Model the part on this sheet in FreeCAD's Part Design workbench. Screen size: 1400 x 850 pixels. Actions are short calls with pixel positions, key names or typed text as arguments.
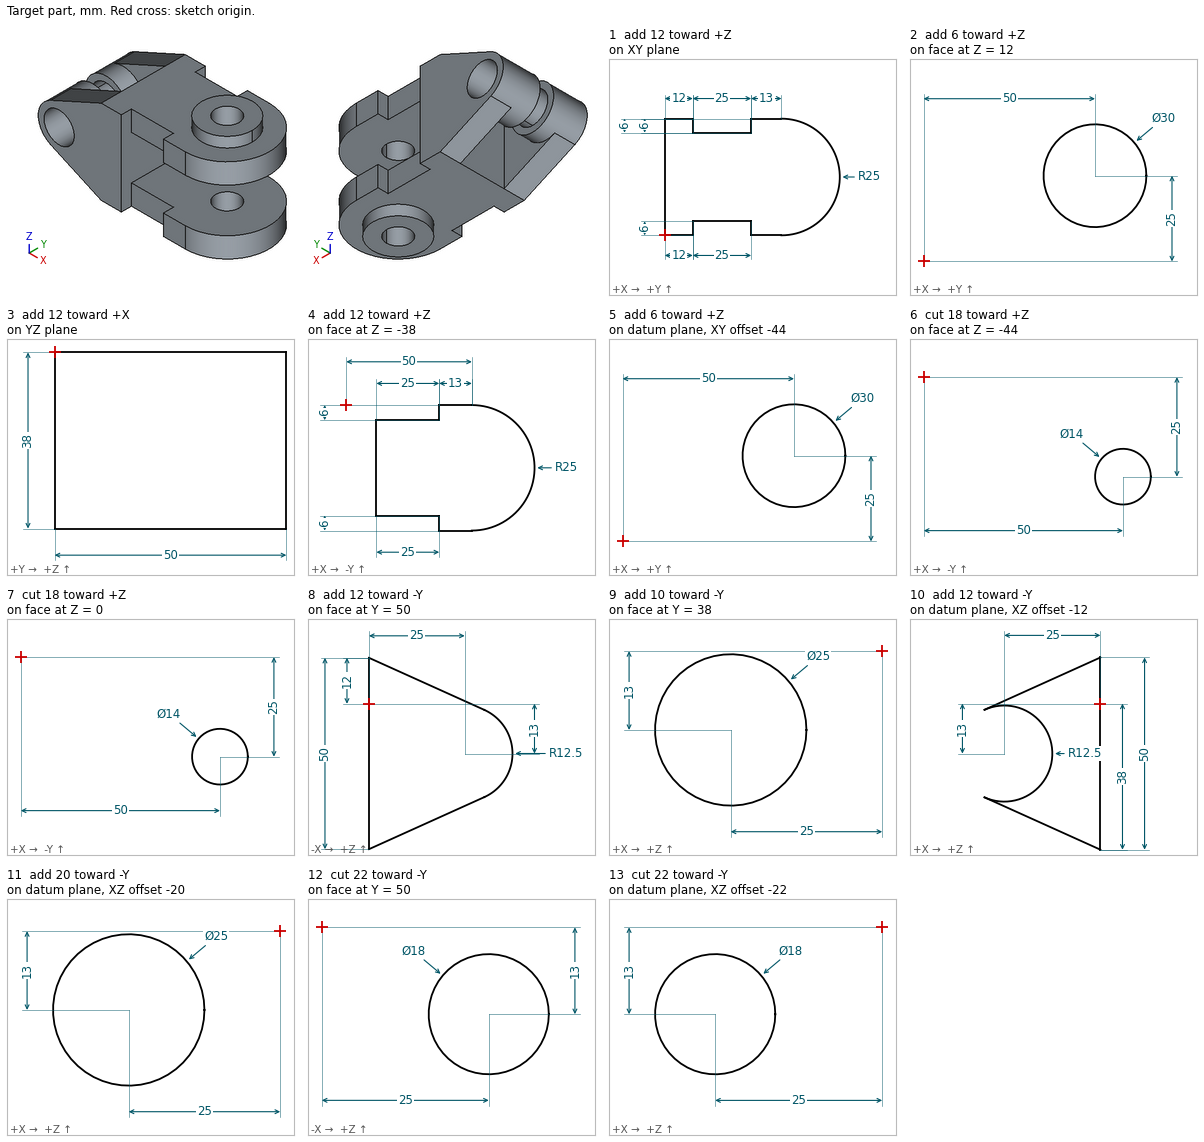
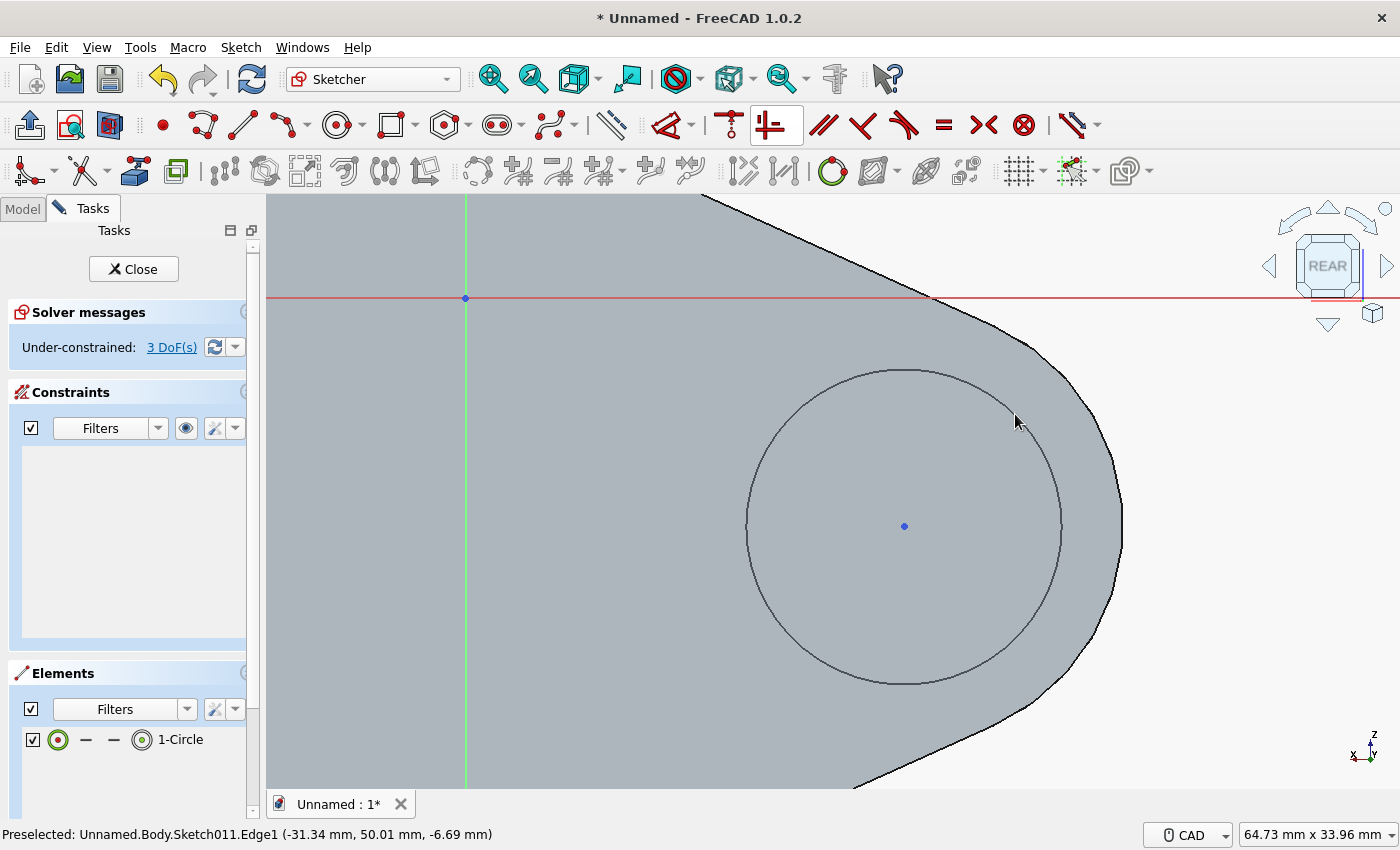
key(d)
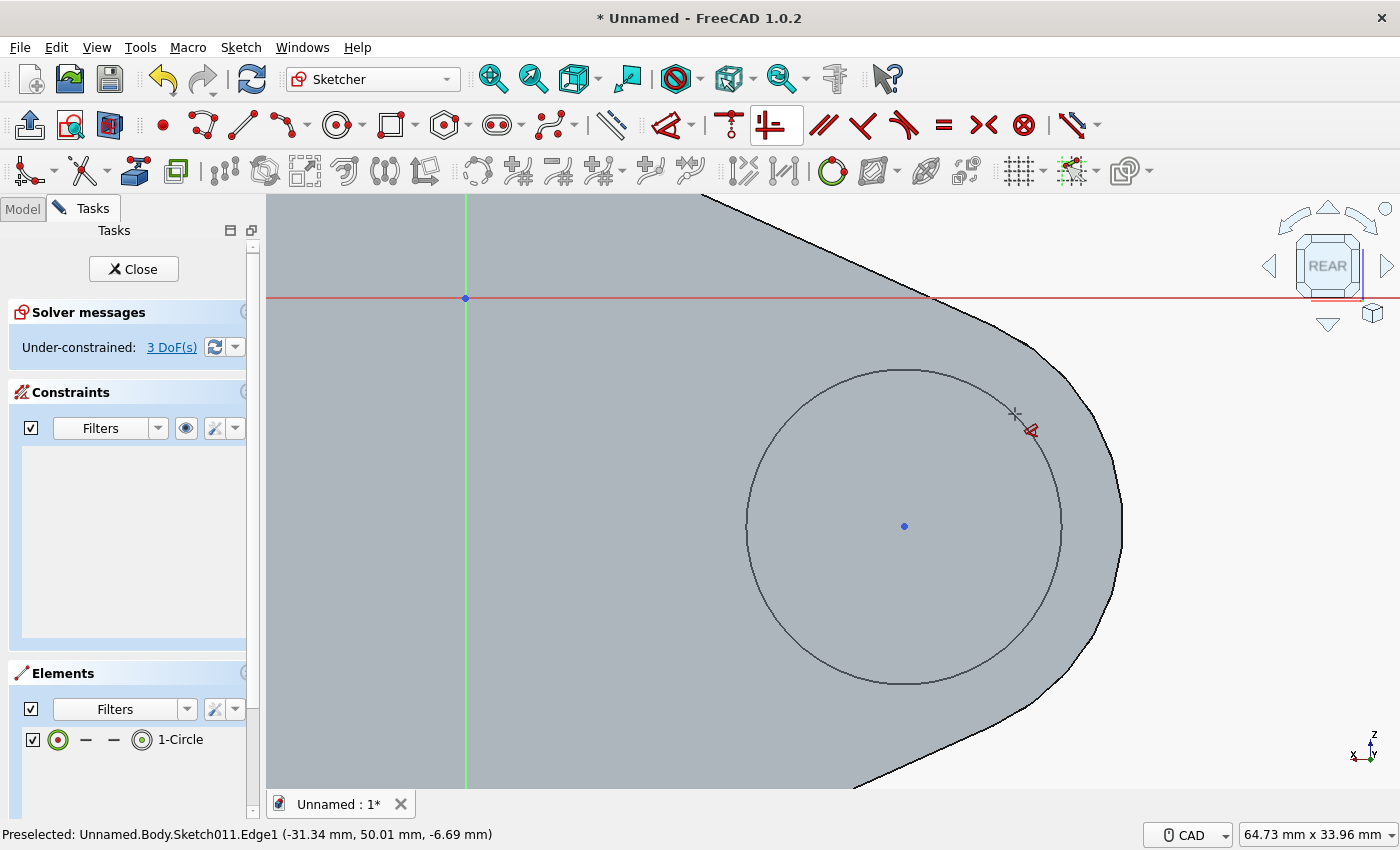
click(1015, 415)
click(1038, 392)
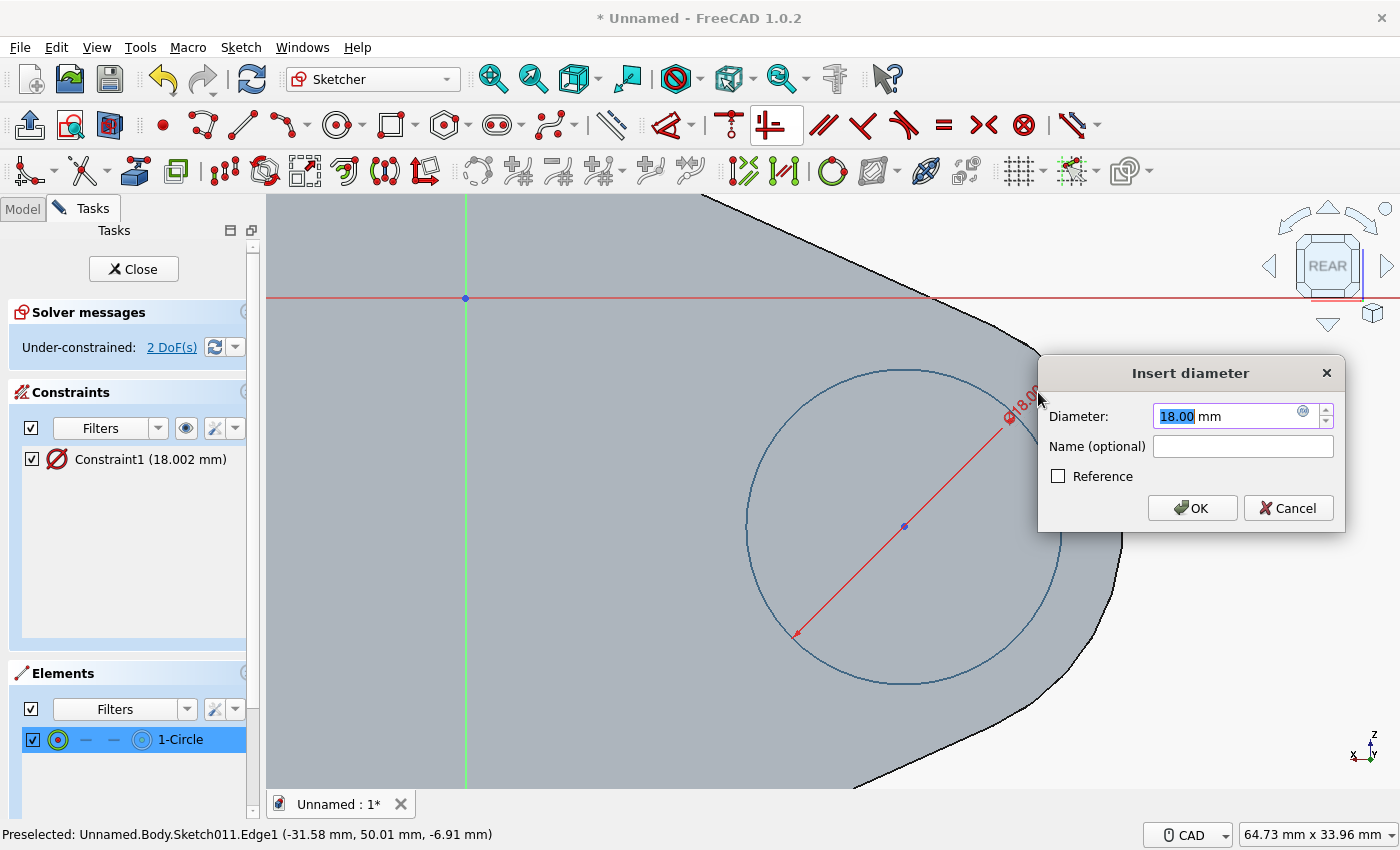
text(18)
key(Return)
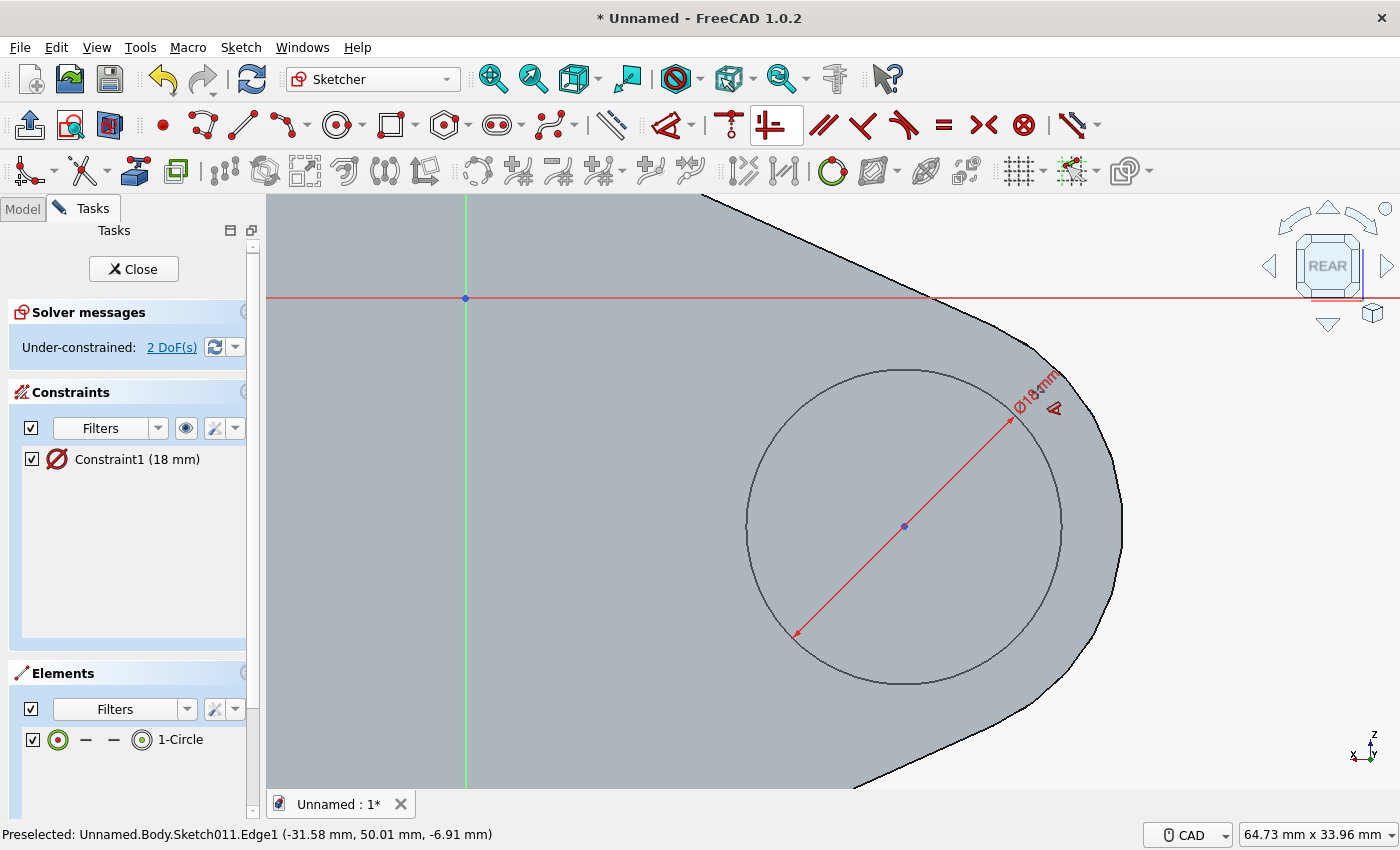
click(904, 527)
click(685, 264)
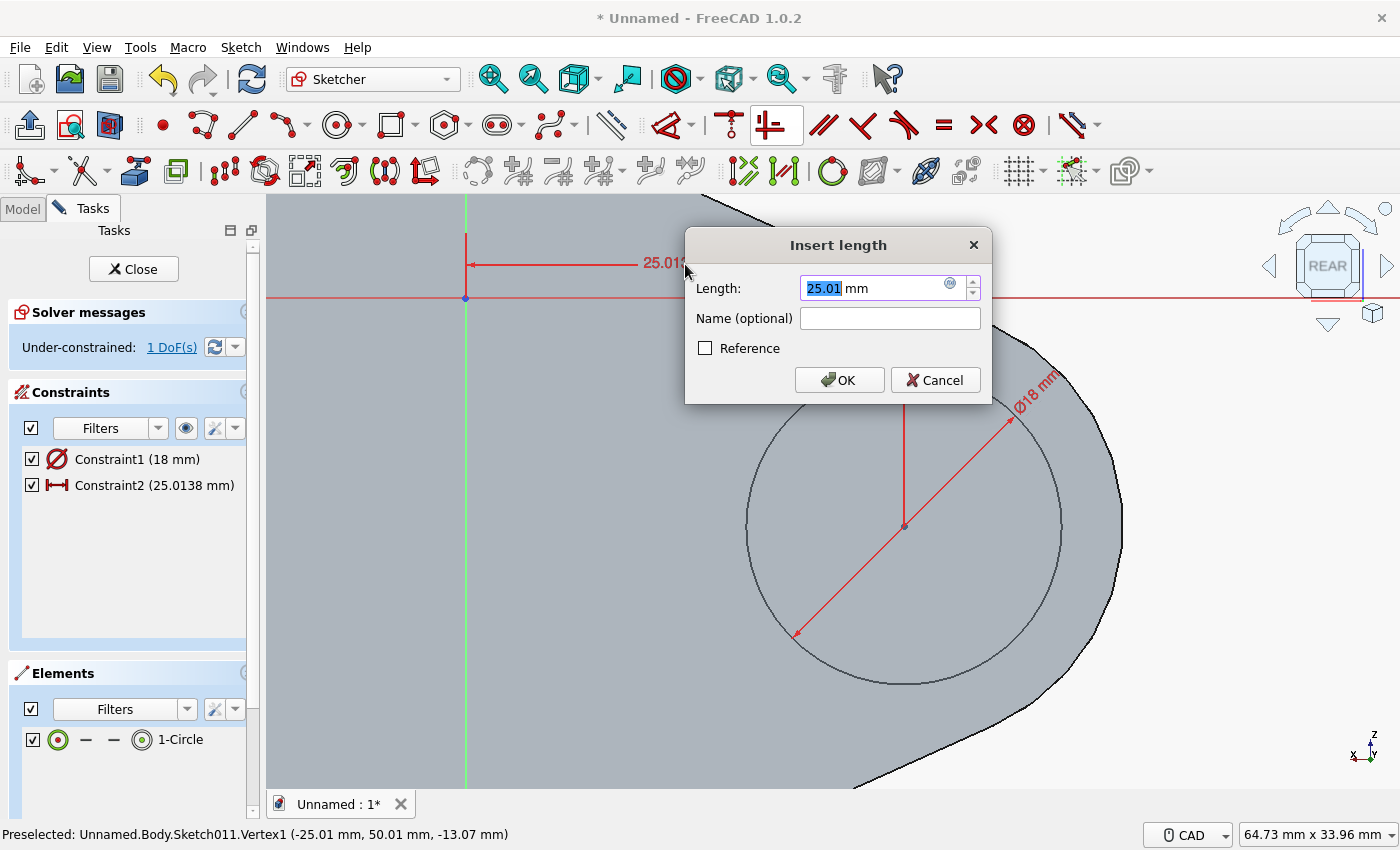
text(25)
key(Return)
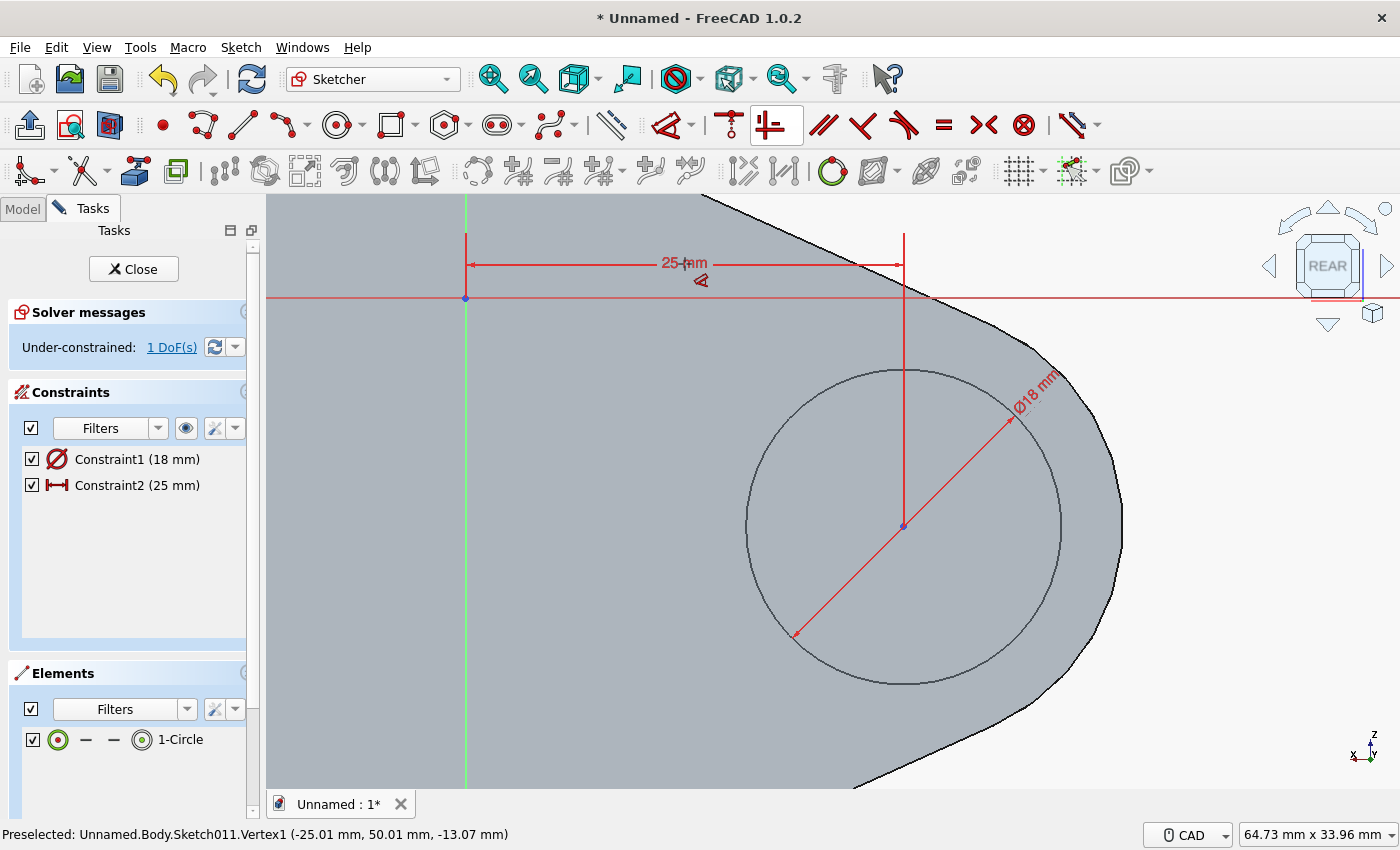
click(904, 527)
click(432, 413)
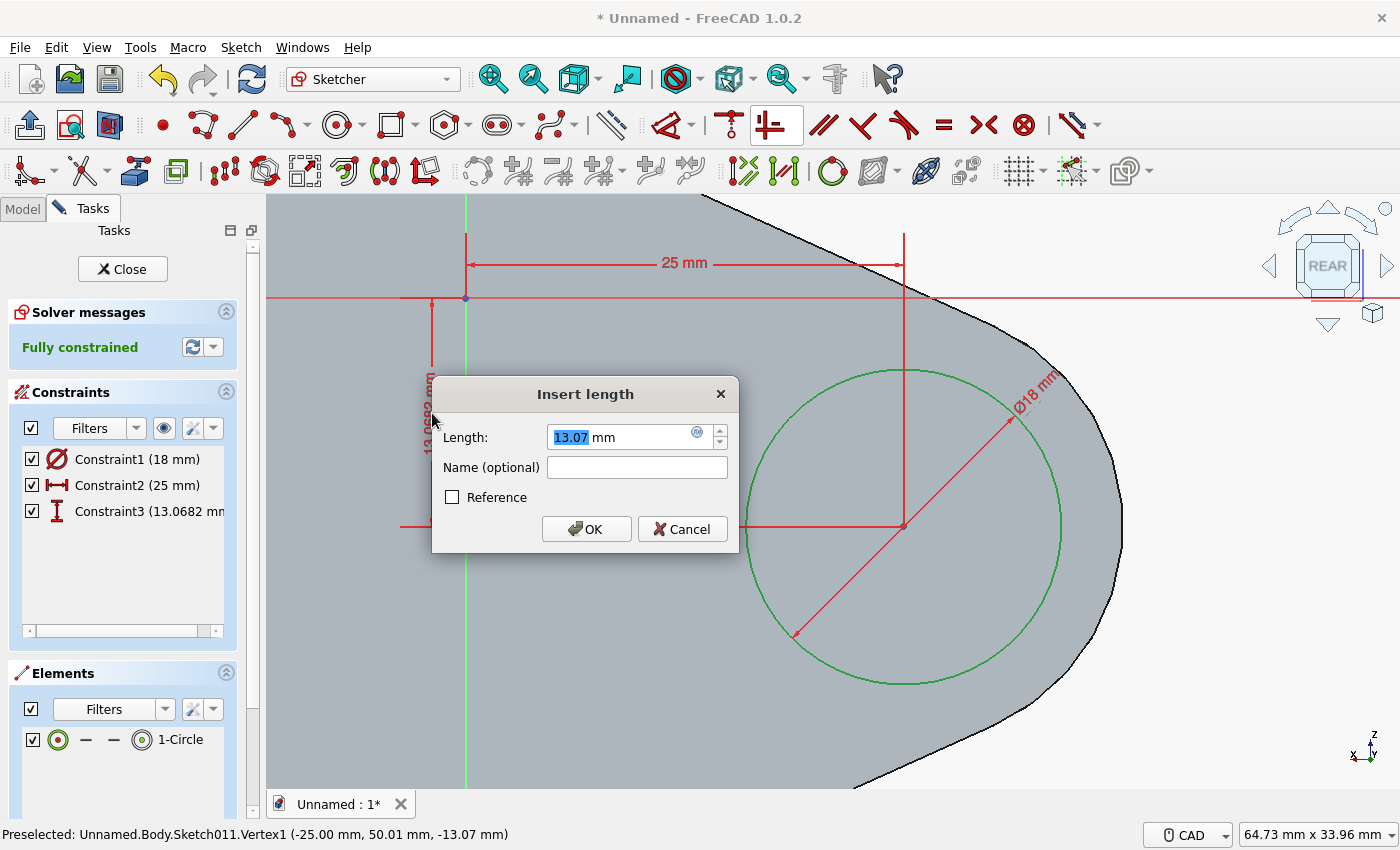
text(13)
key(Return)
key(Escape)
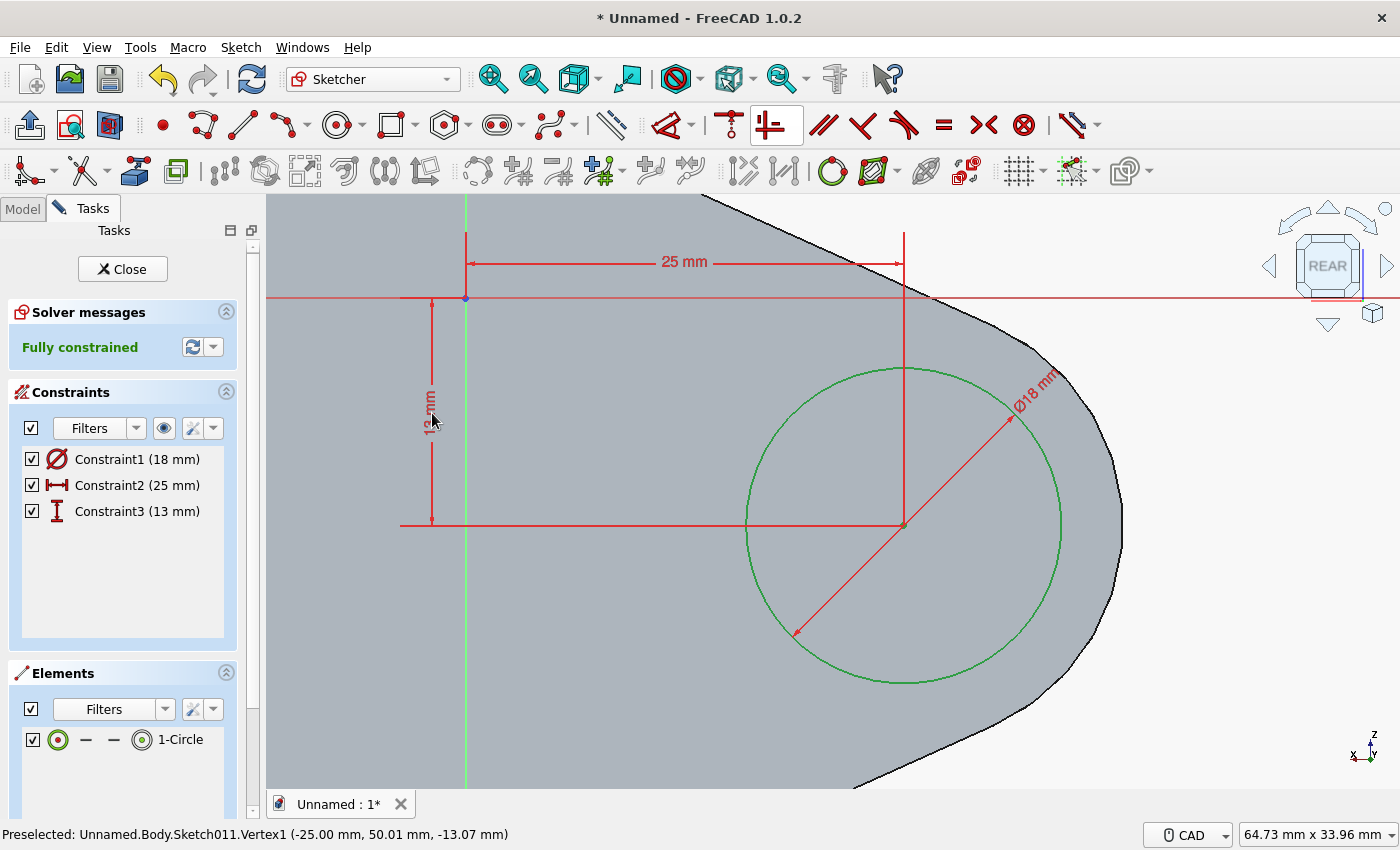
click(123, 269)